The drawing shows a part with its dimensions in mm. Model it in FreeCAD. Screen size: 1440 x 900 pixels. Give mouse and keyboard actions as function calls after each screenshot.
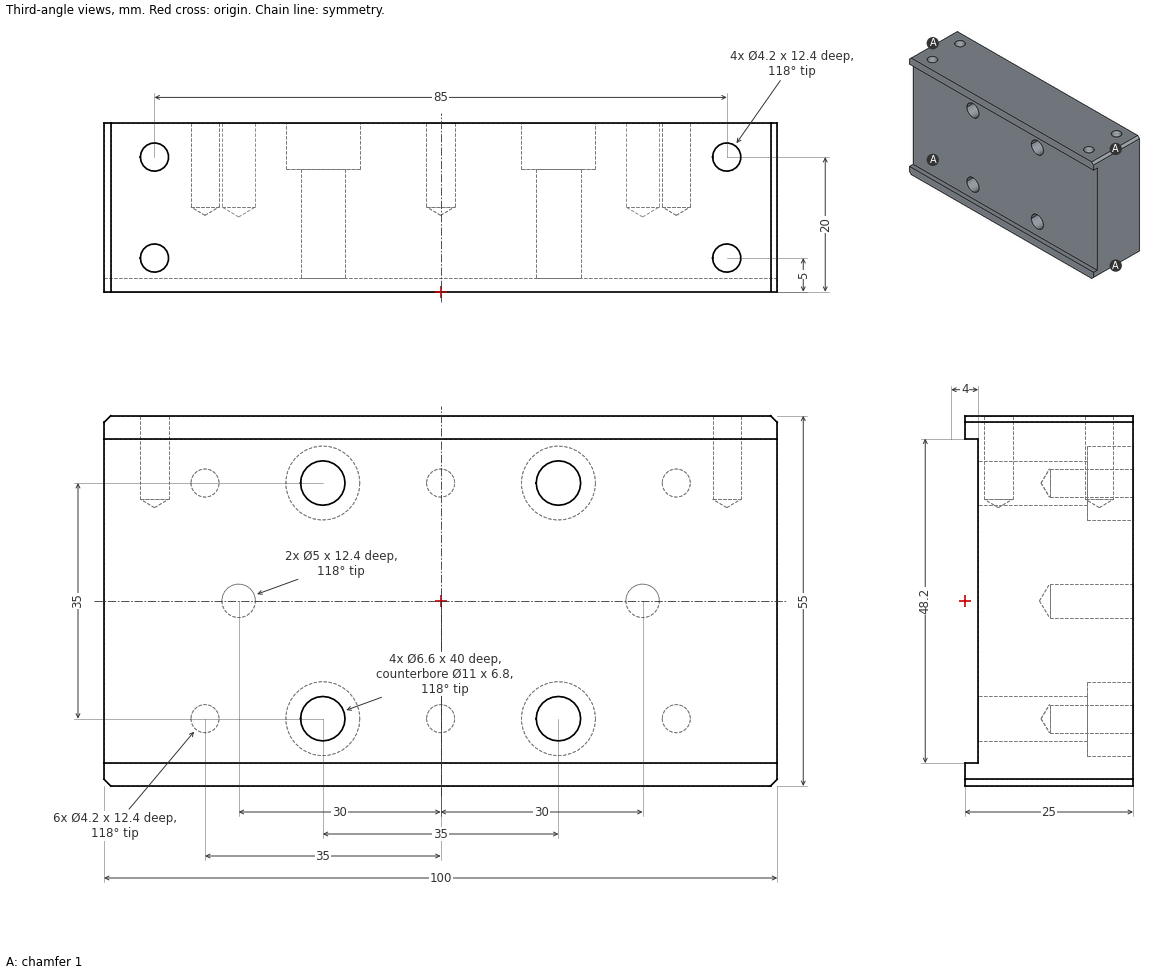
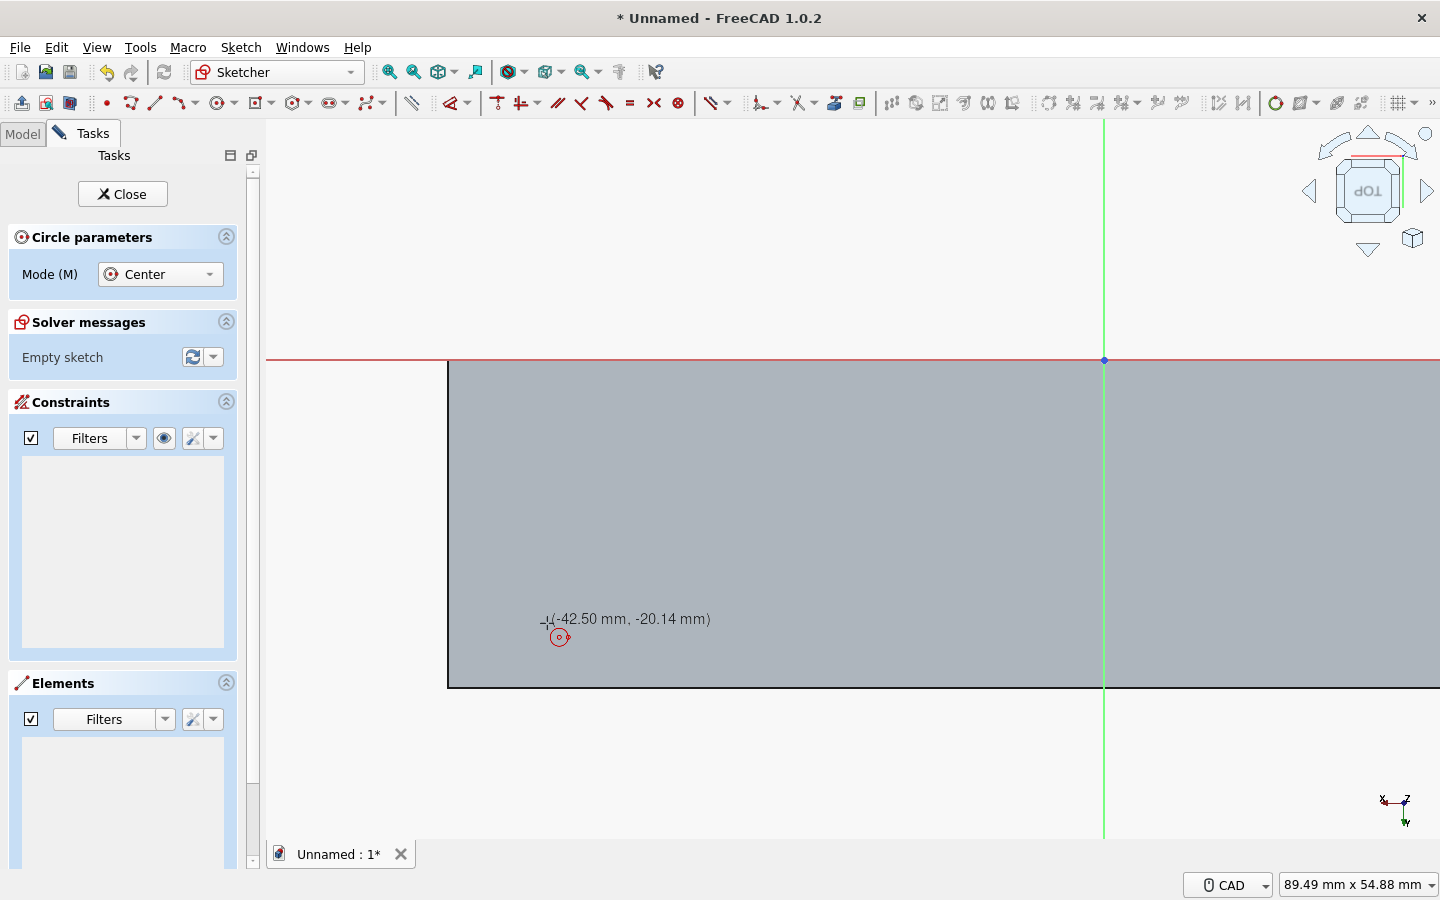
click(547, 622)
move(566, 603)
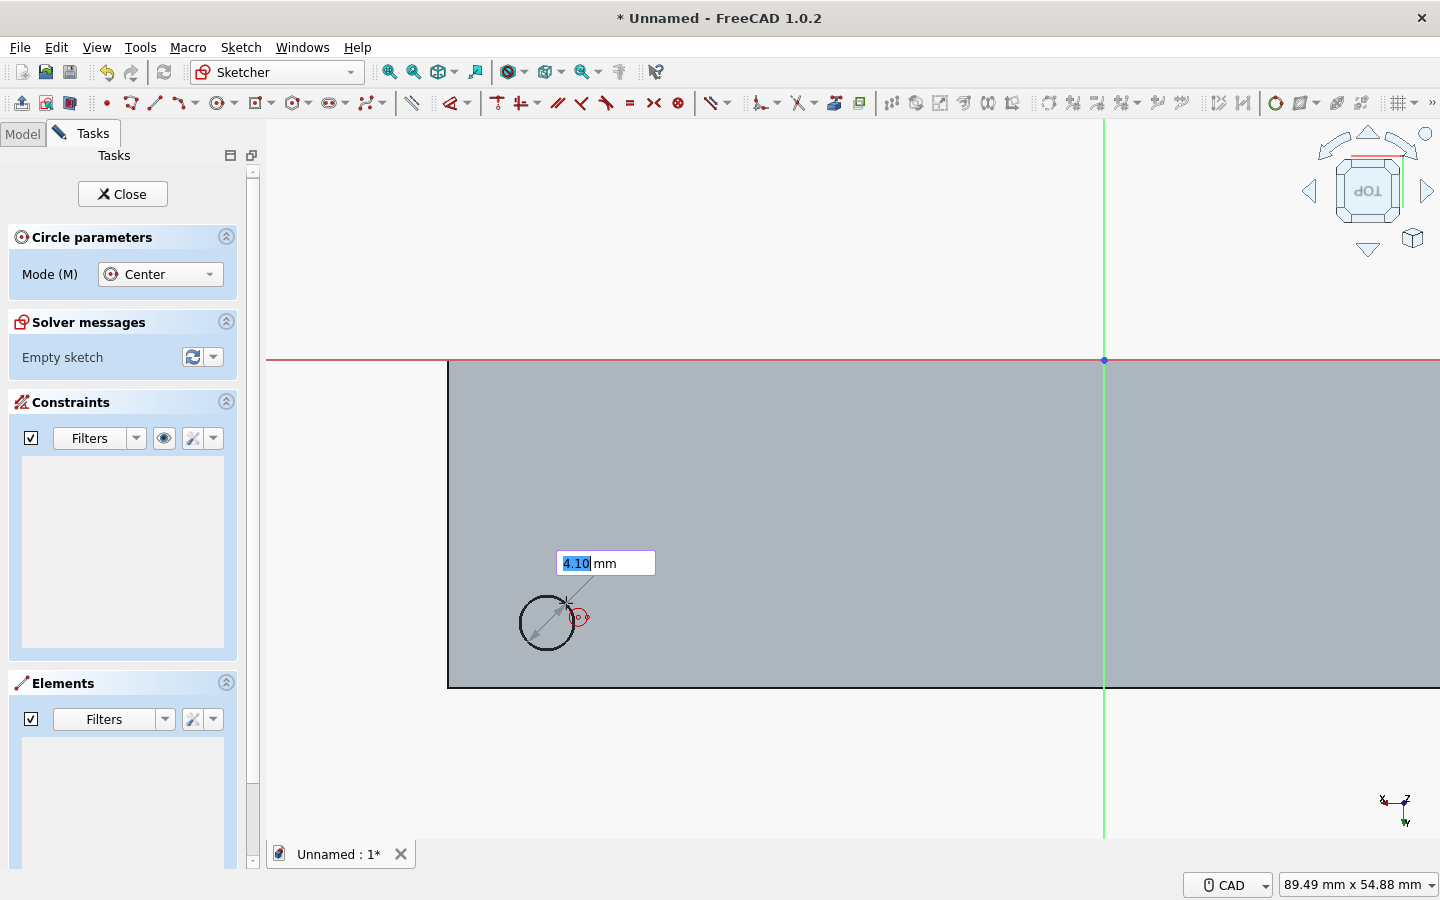
text(4.2)
key(Return)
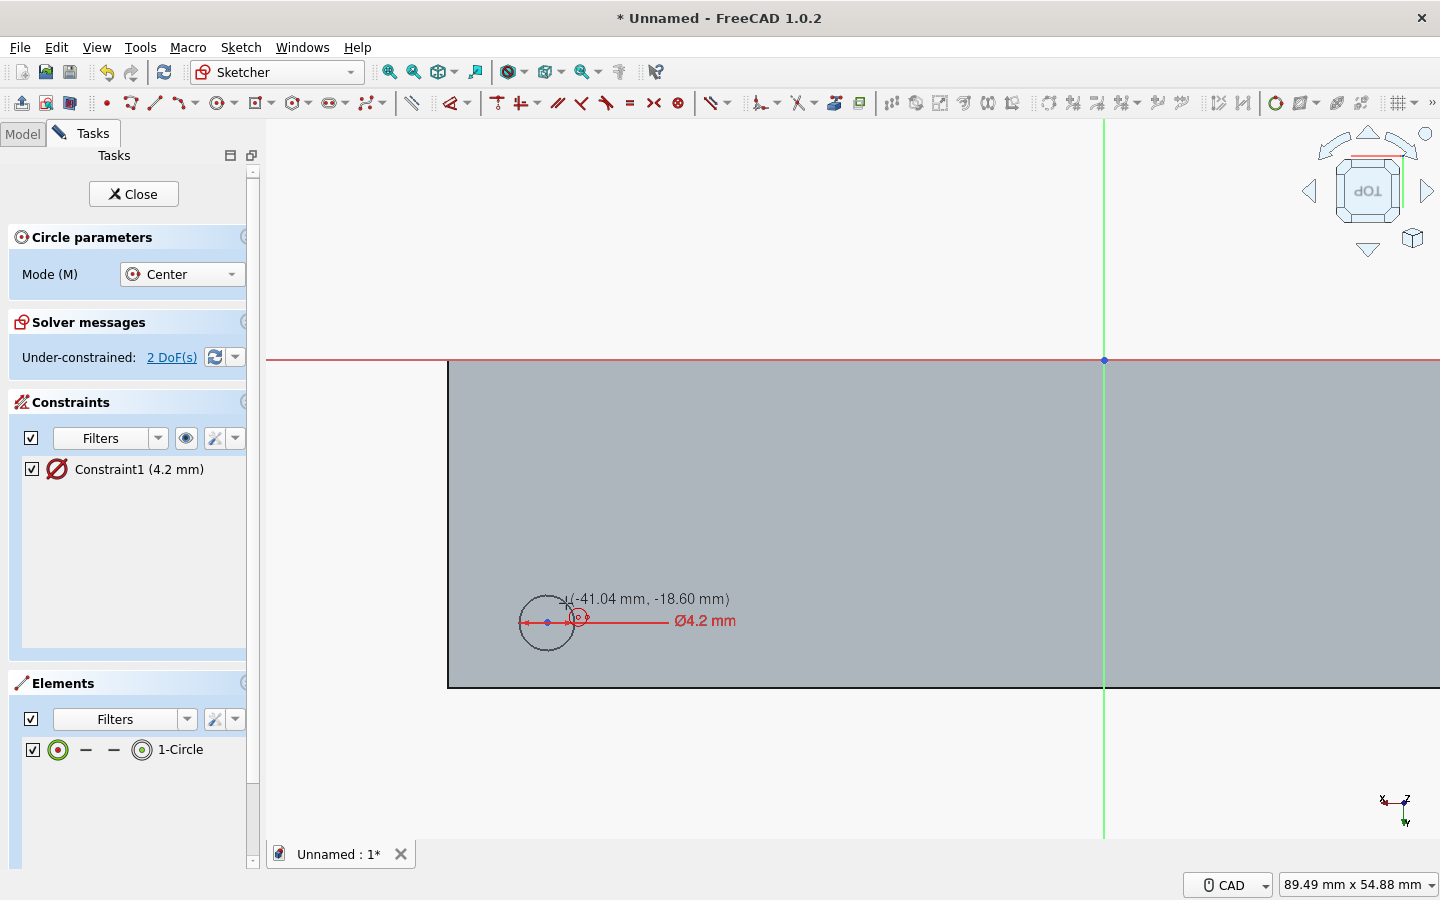
click(547, 426)
move(566, 406)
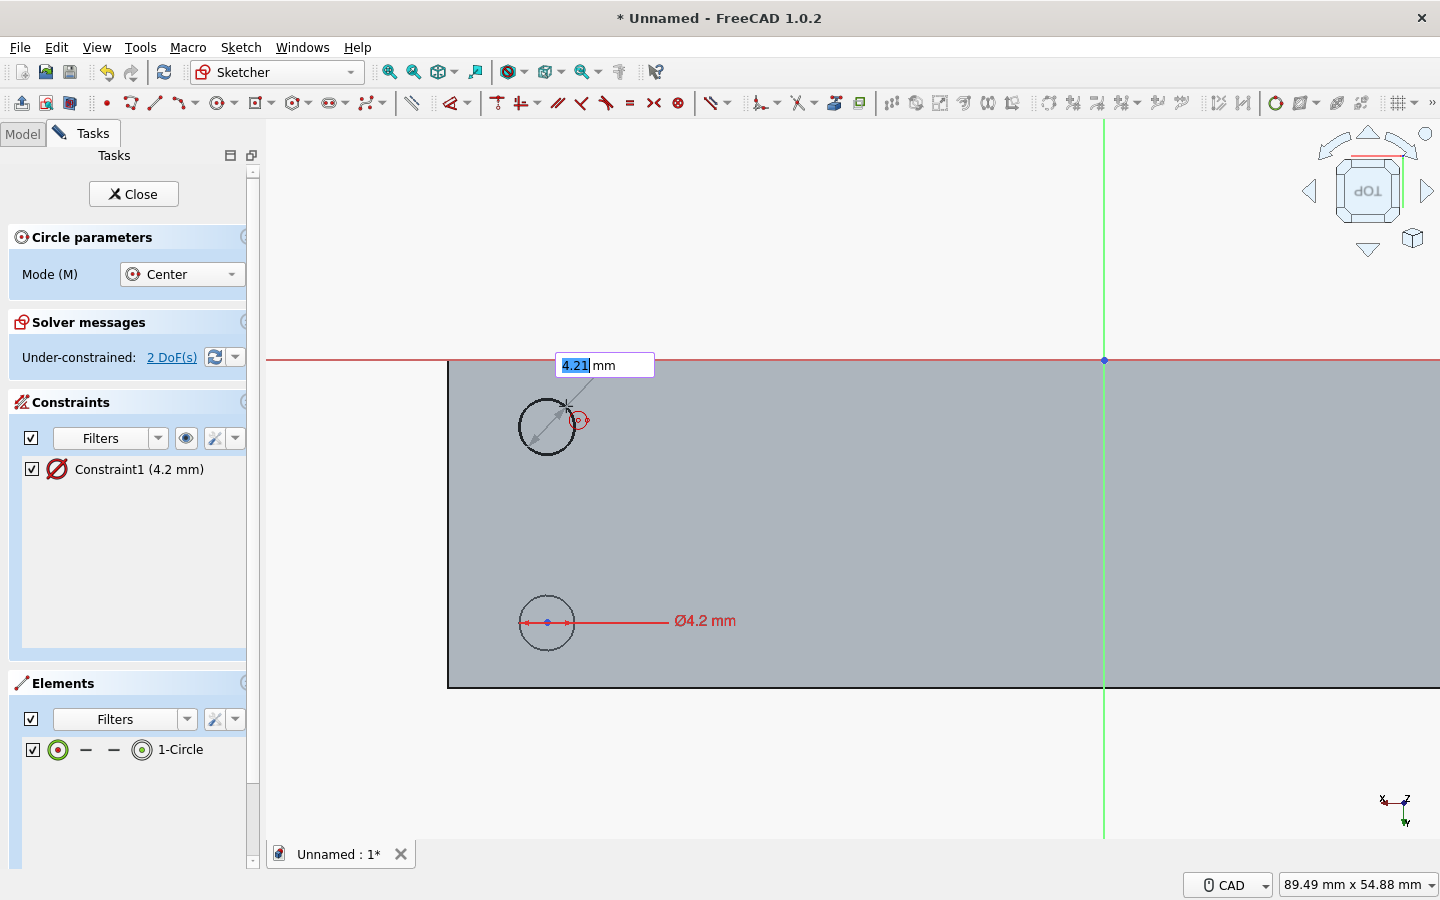
text(4.2)
key(Return)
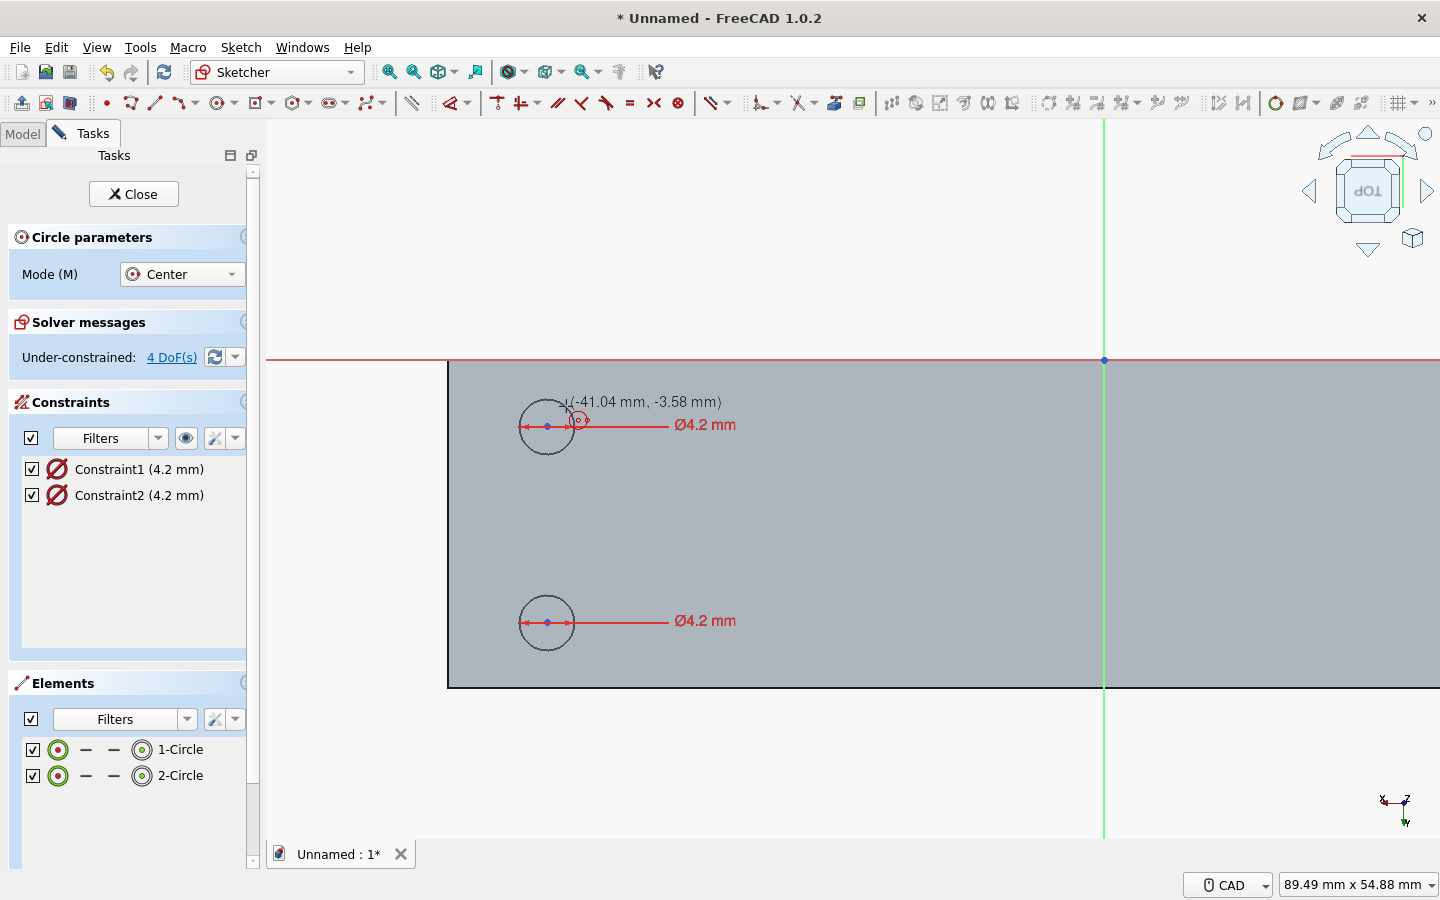
scroll(395, 447, down, 3)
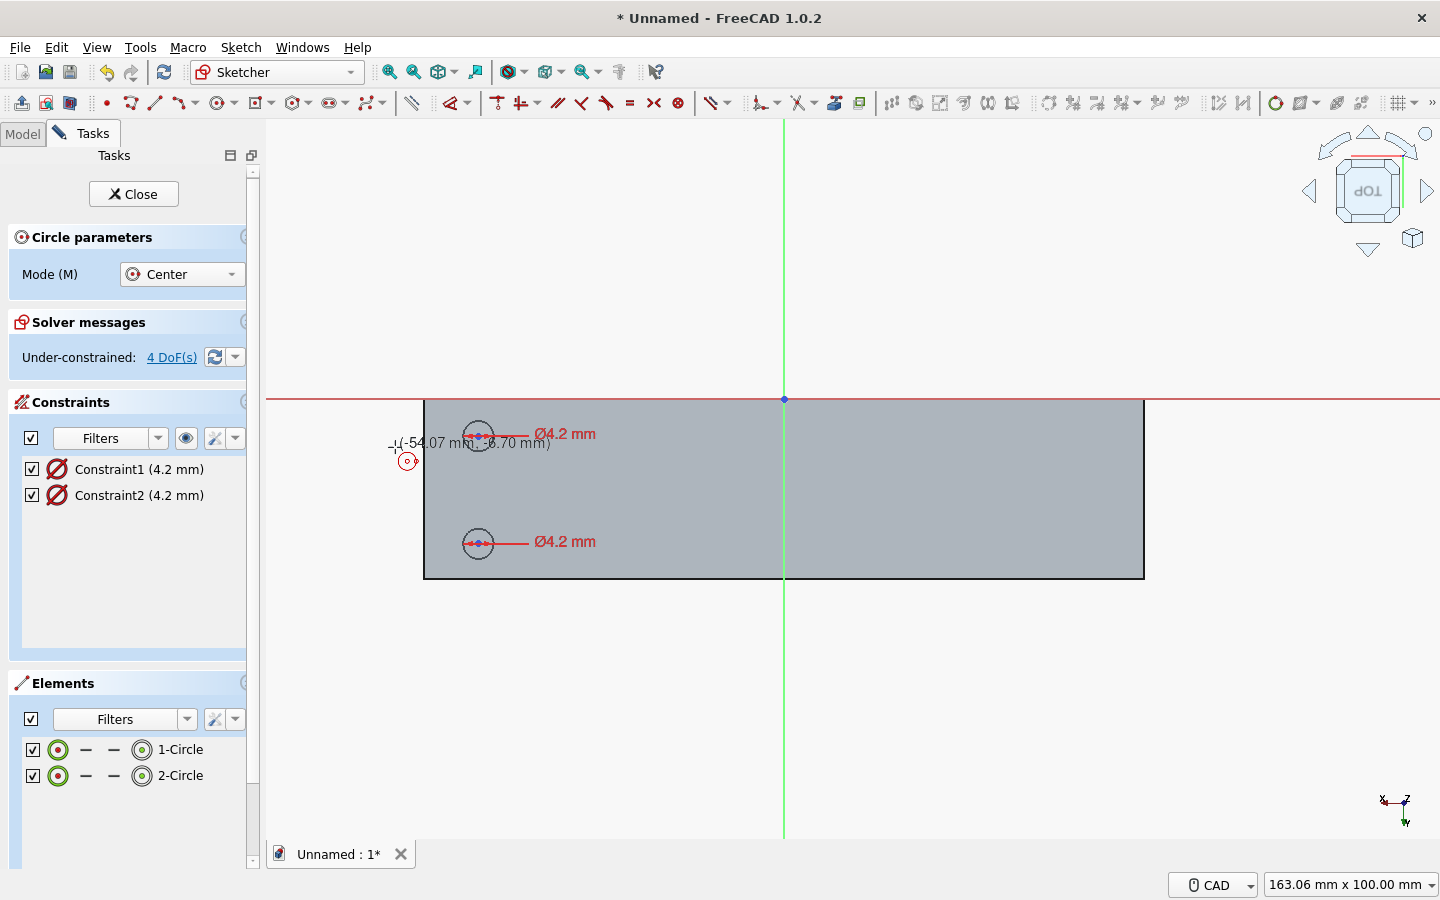
scroll(1090, 543, up, 3)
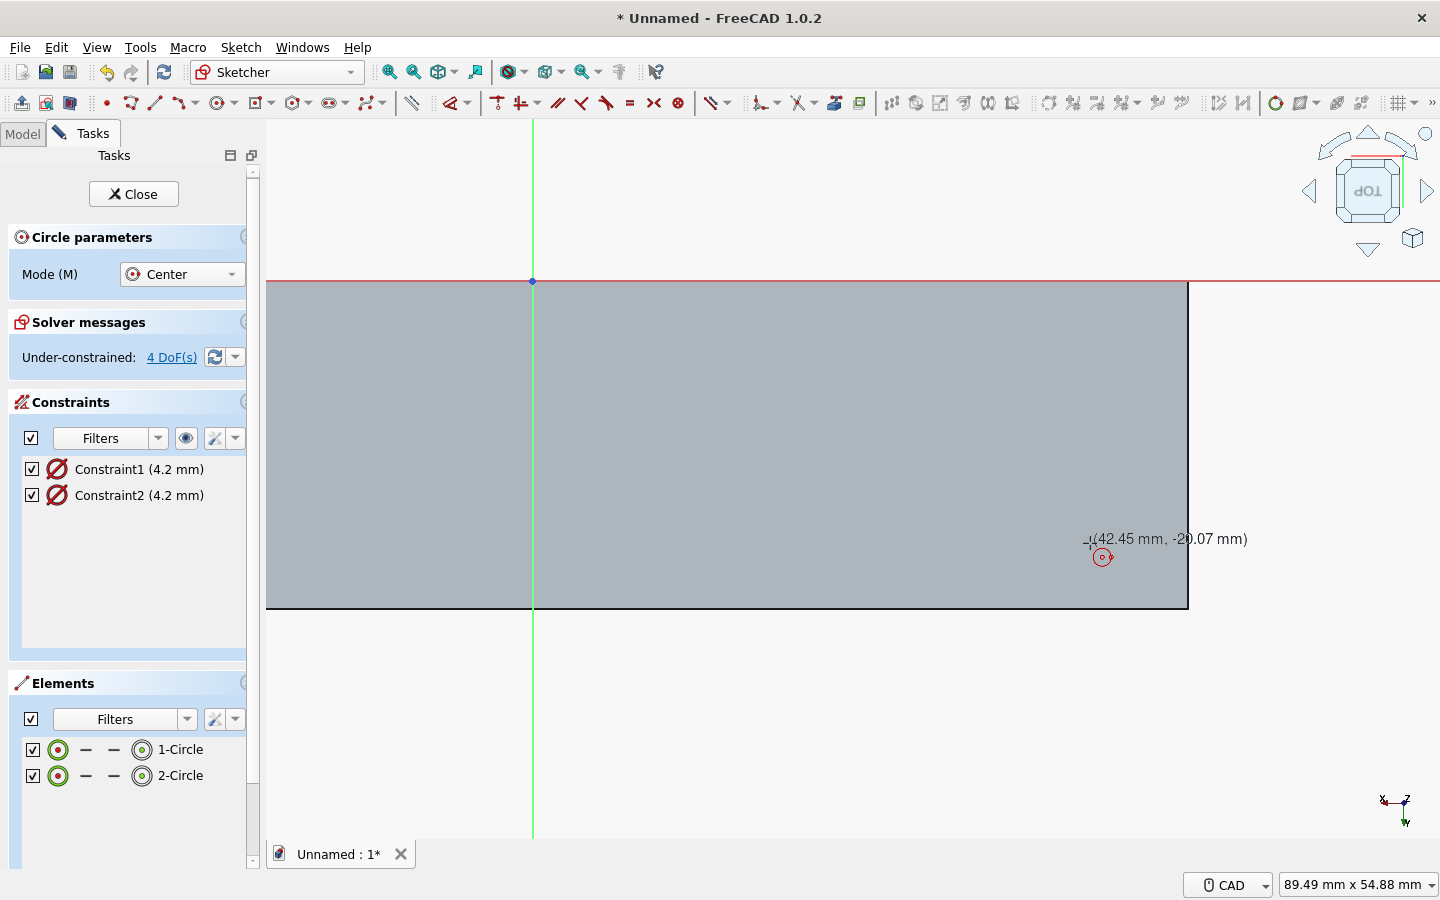
click(1090, 543)
move(1110, 524)